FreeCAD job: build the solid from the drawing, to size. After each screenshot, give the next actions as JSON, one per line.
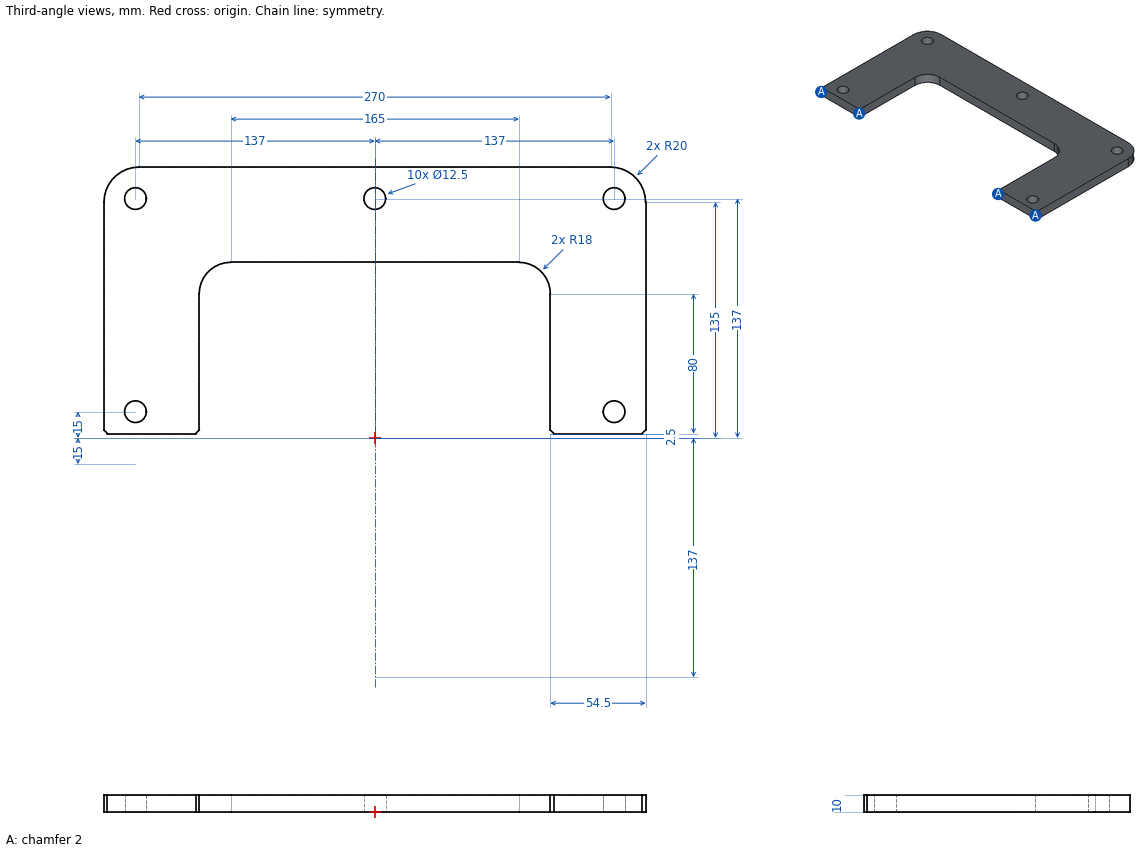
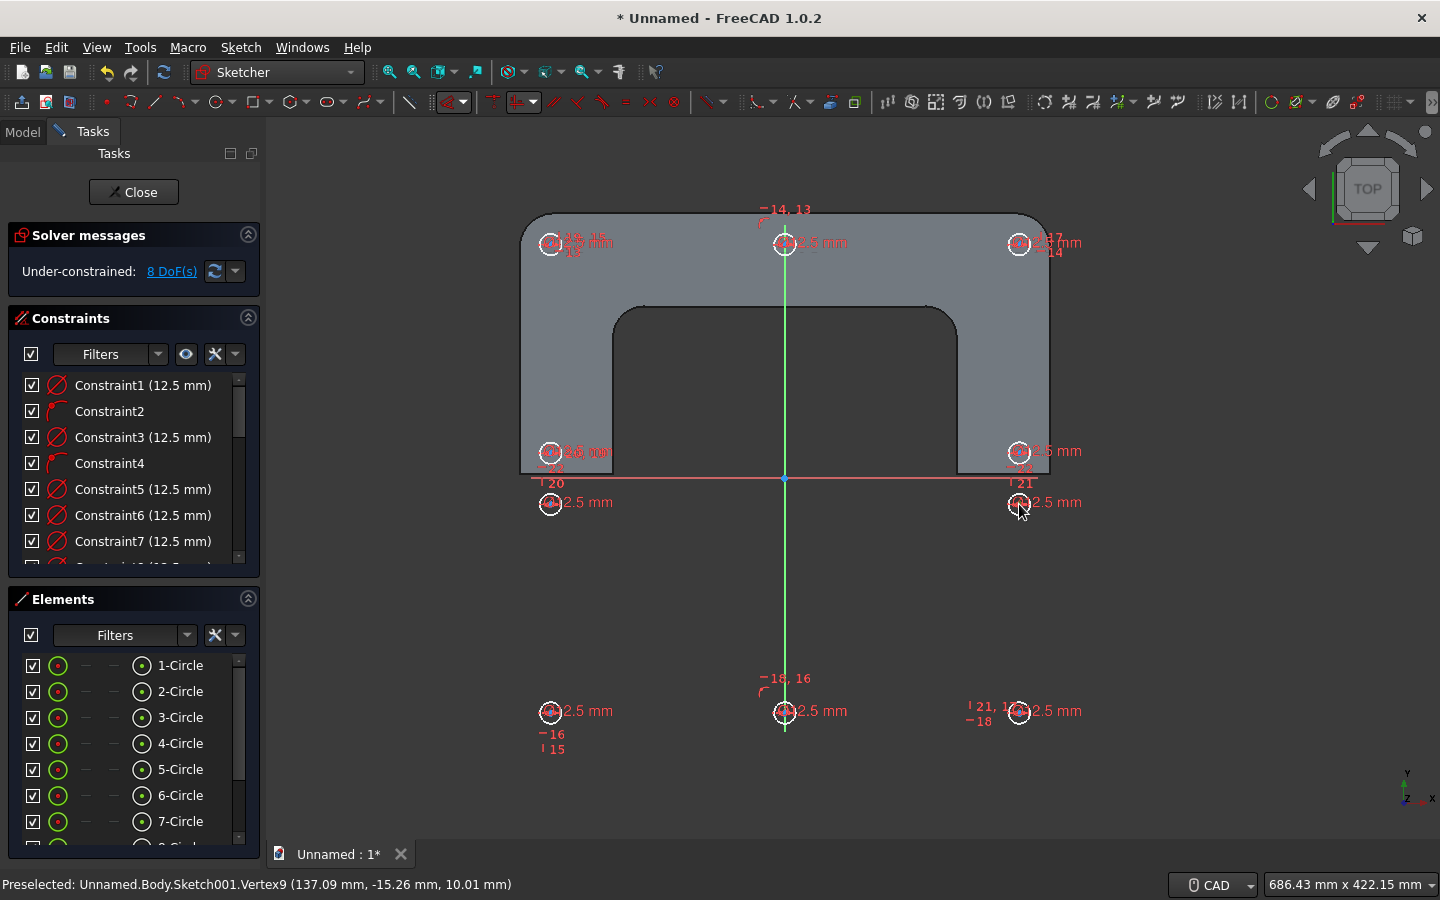
{"action": "left_click", "coordinate": [1019, 453]}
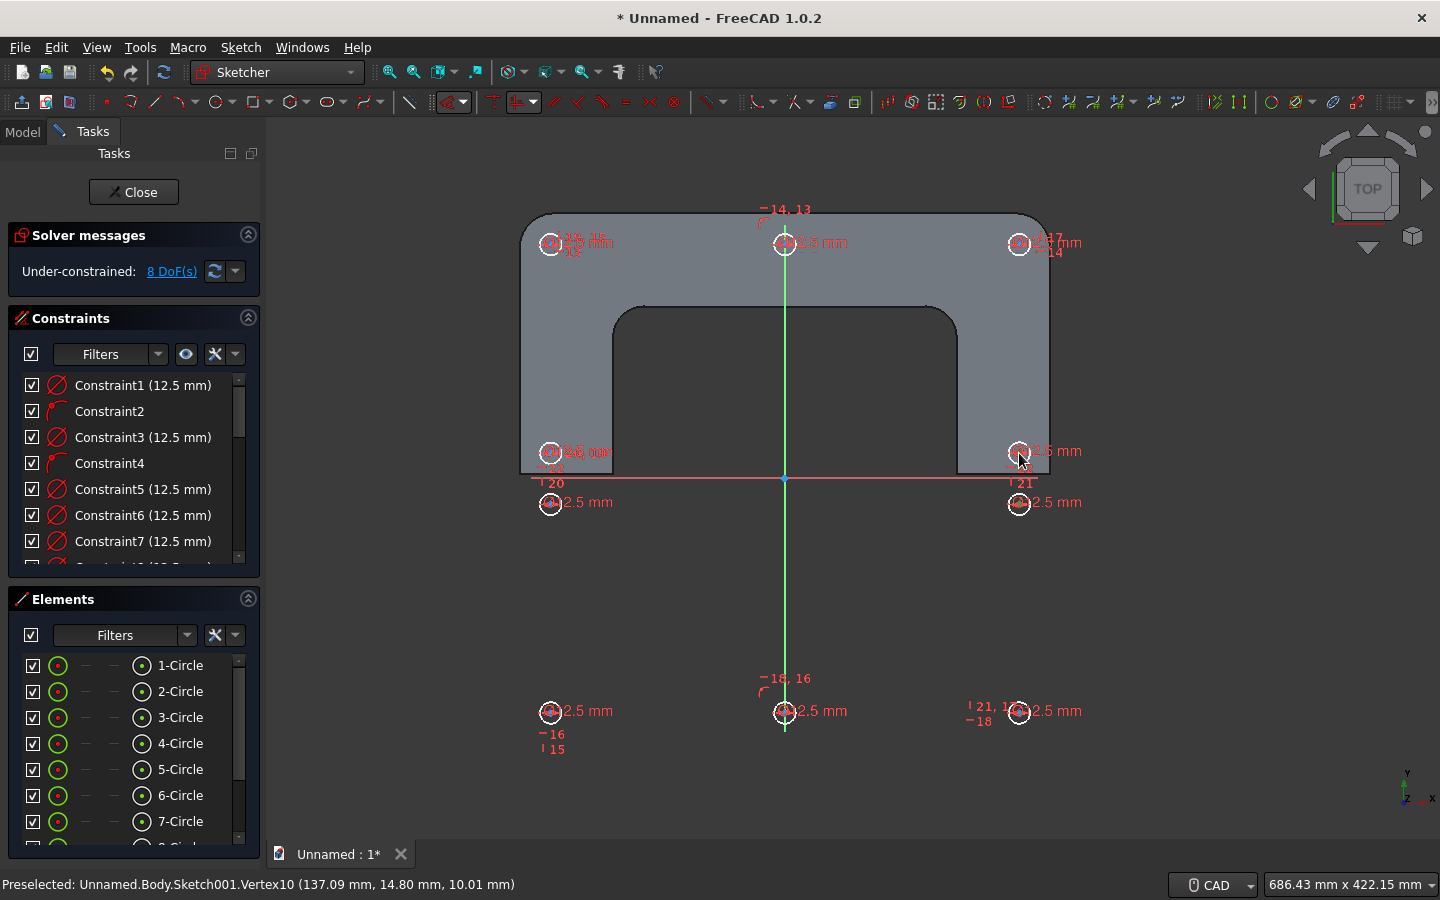
{"action": "key", "text": "v"}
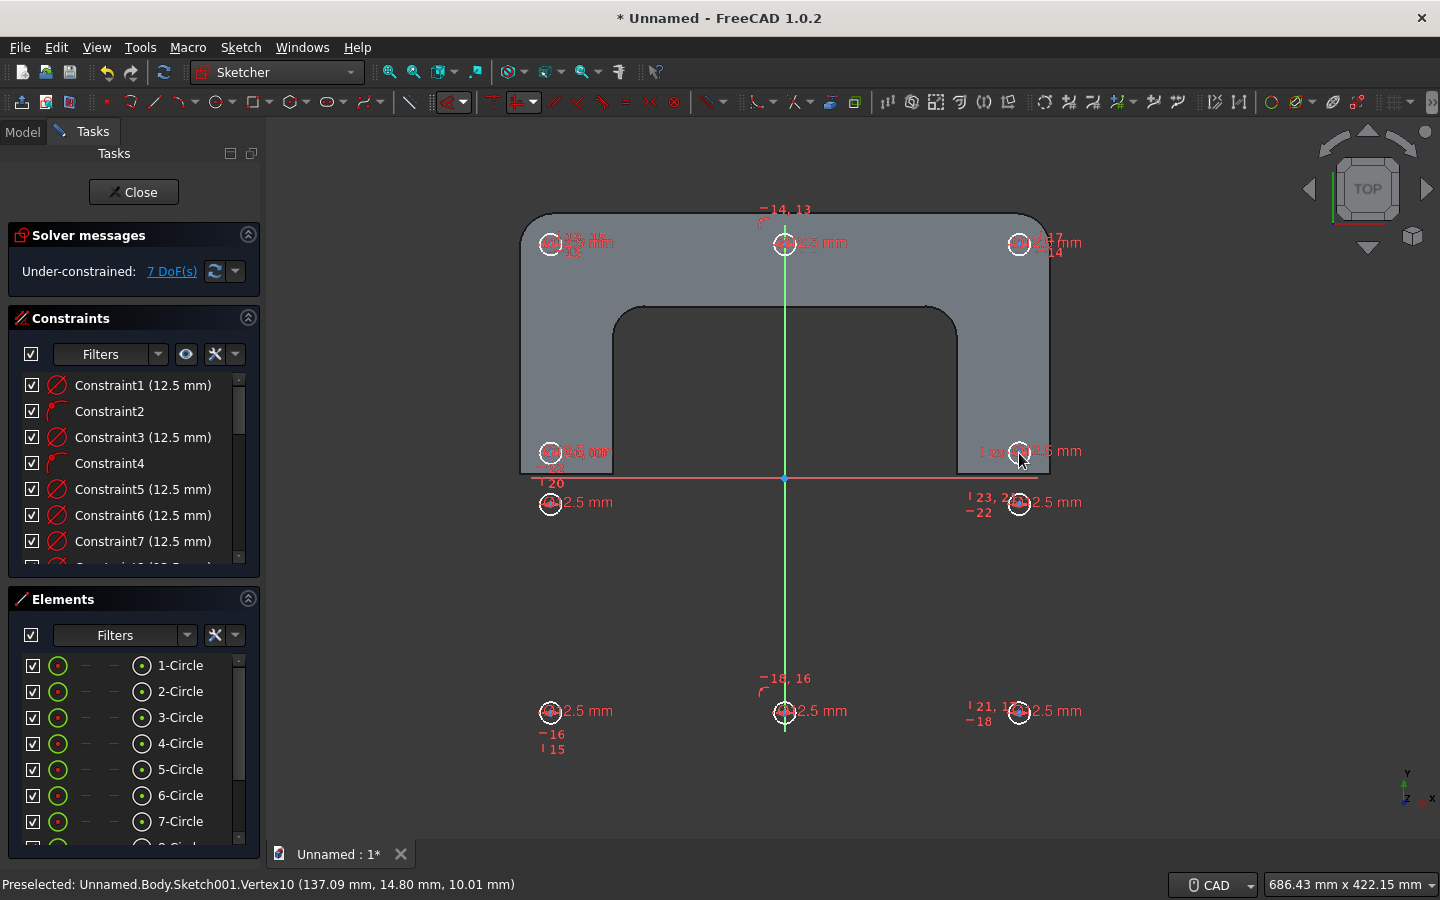
{"action": "left_click", "coordinate": [551, 453]}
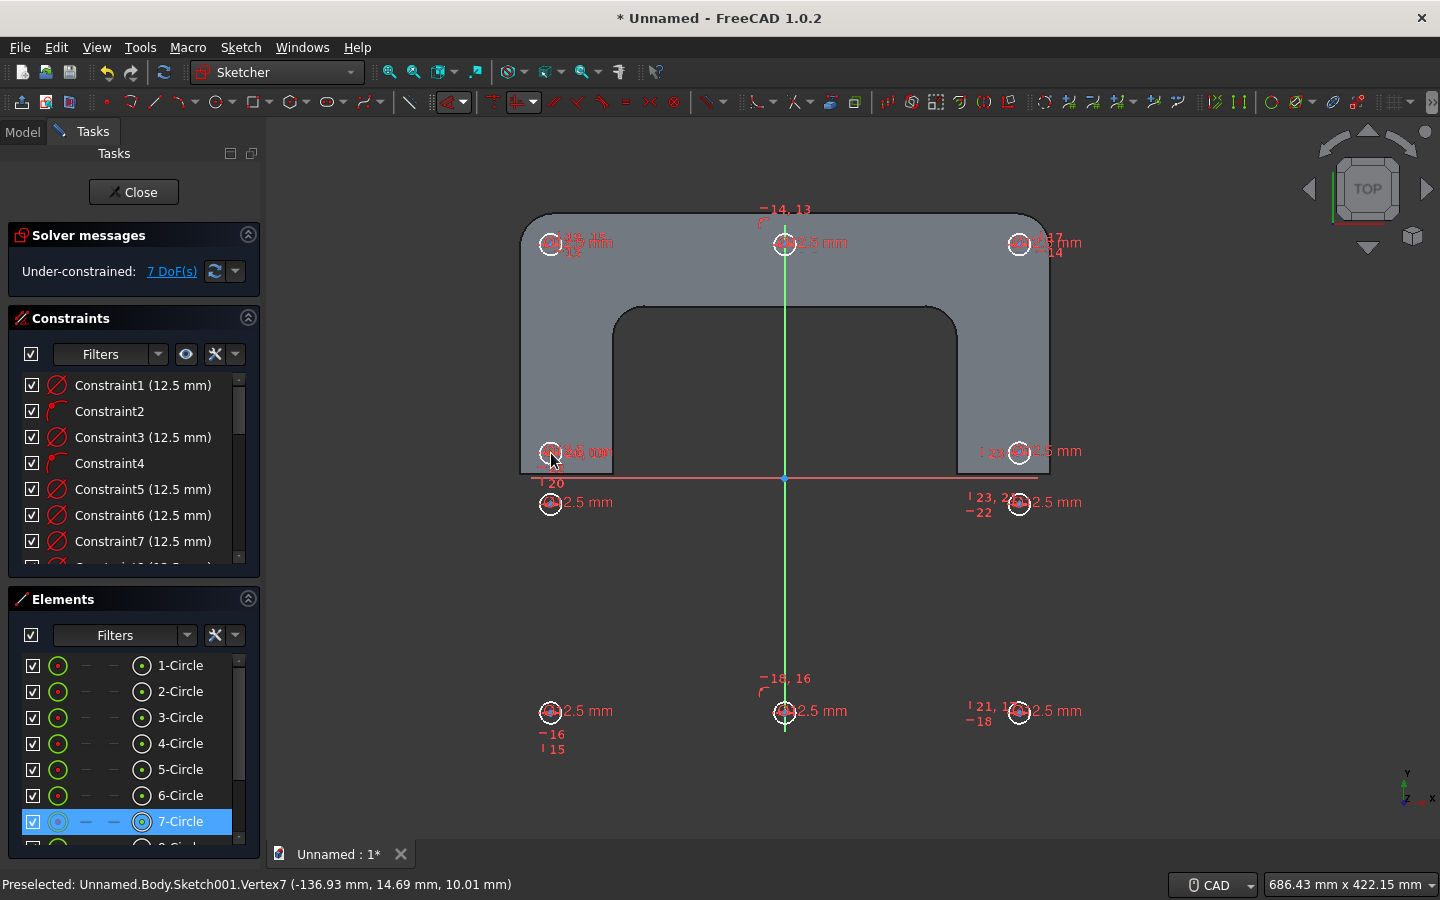
{"action": "left_click", "coordinate": [1019, 453]}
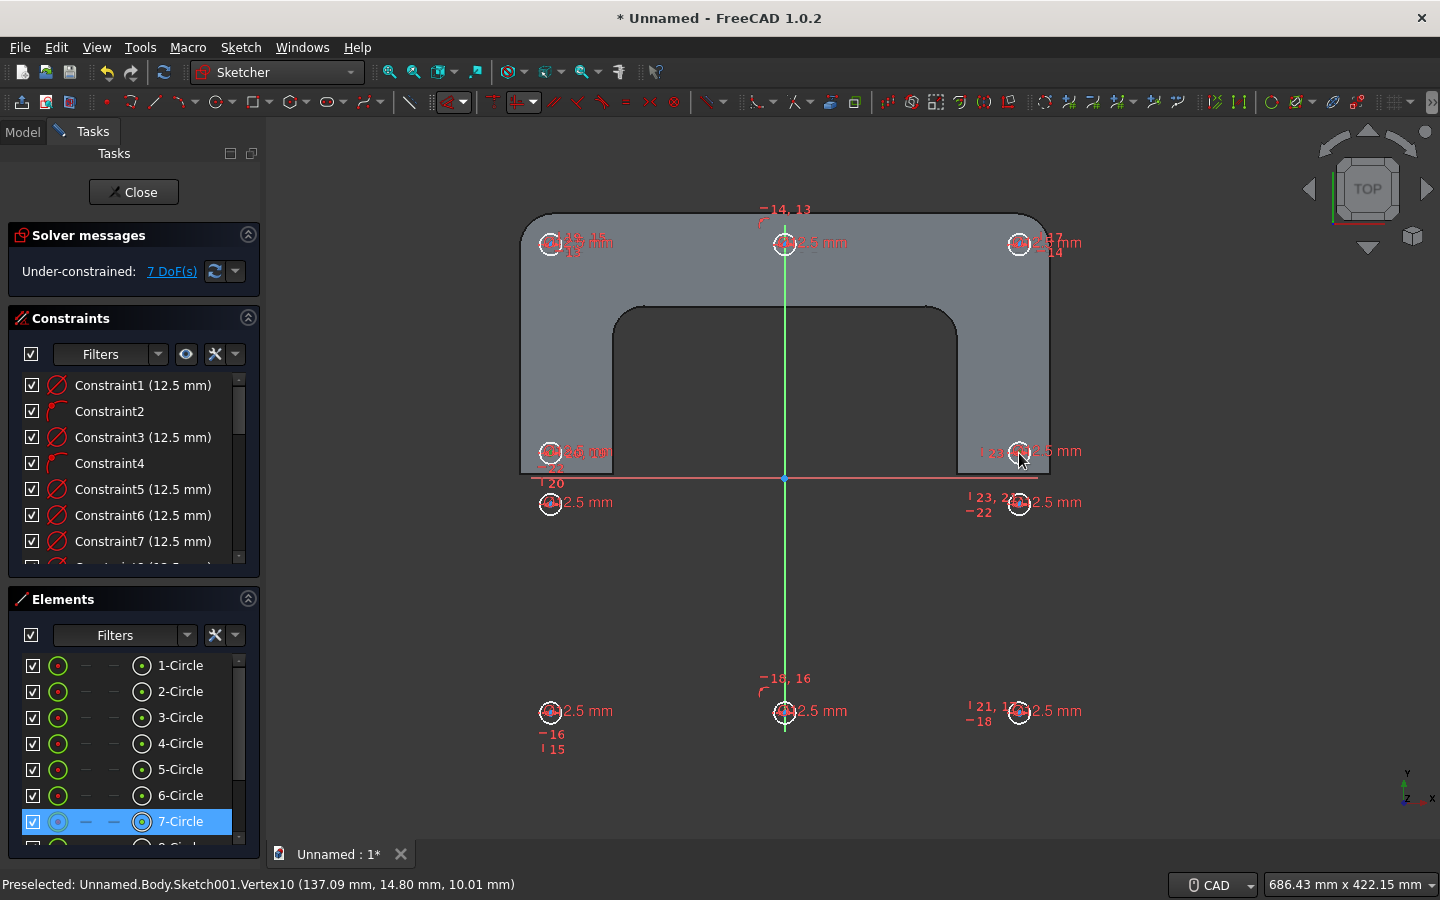
{"action": "key", "text": "h"}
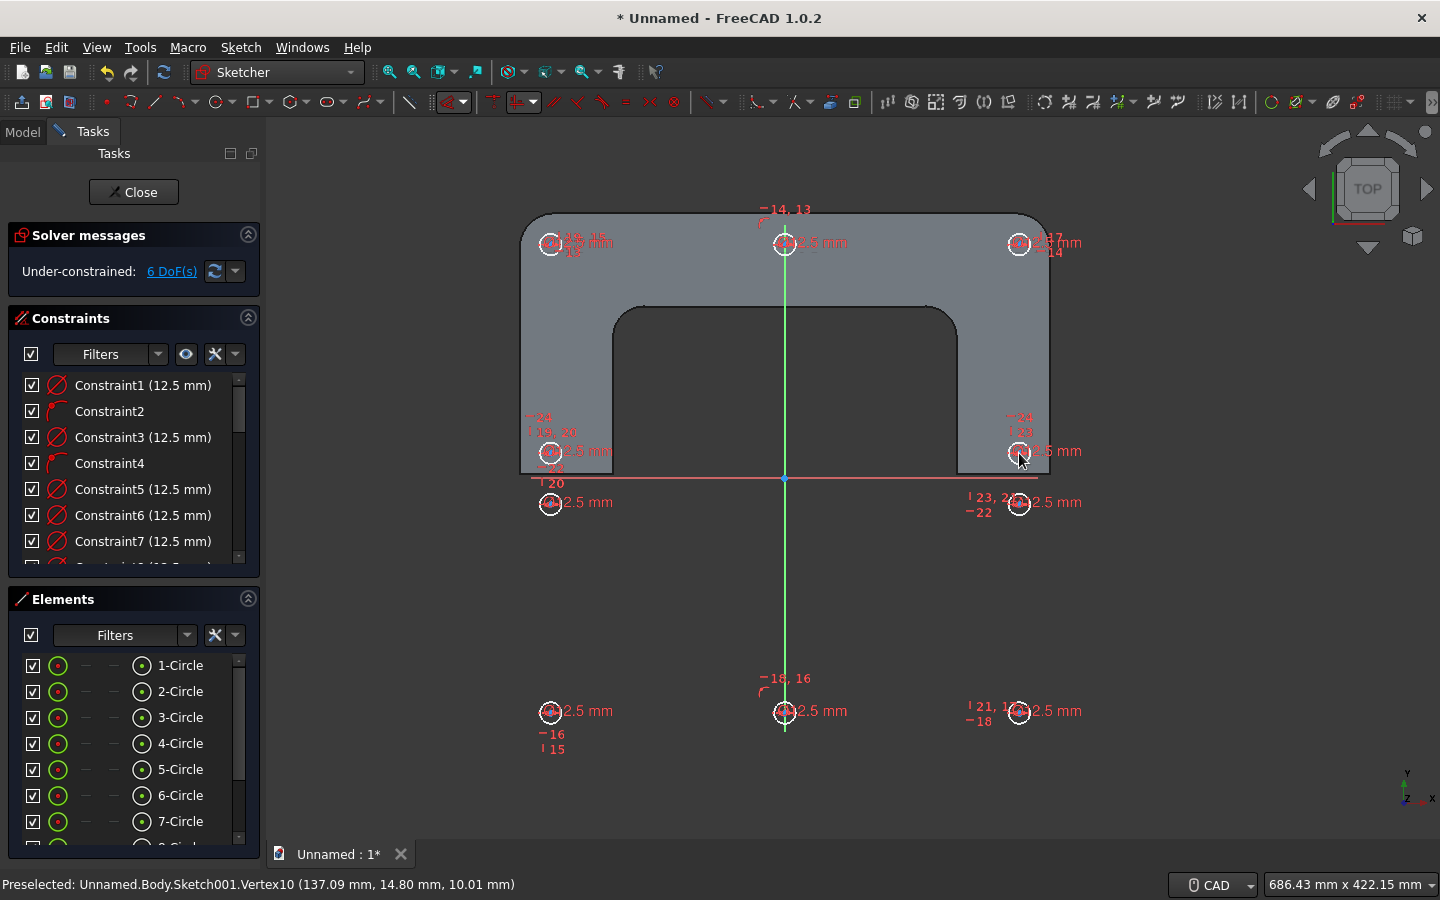
{"action": "scroll", "coordinate": [551, 453], "scroll_direction": "up", "scroll_amount": 3}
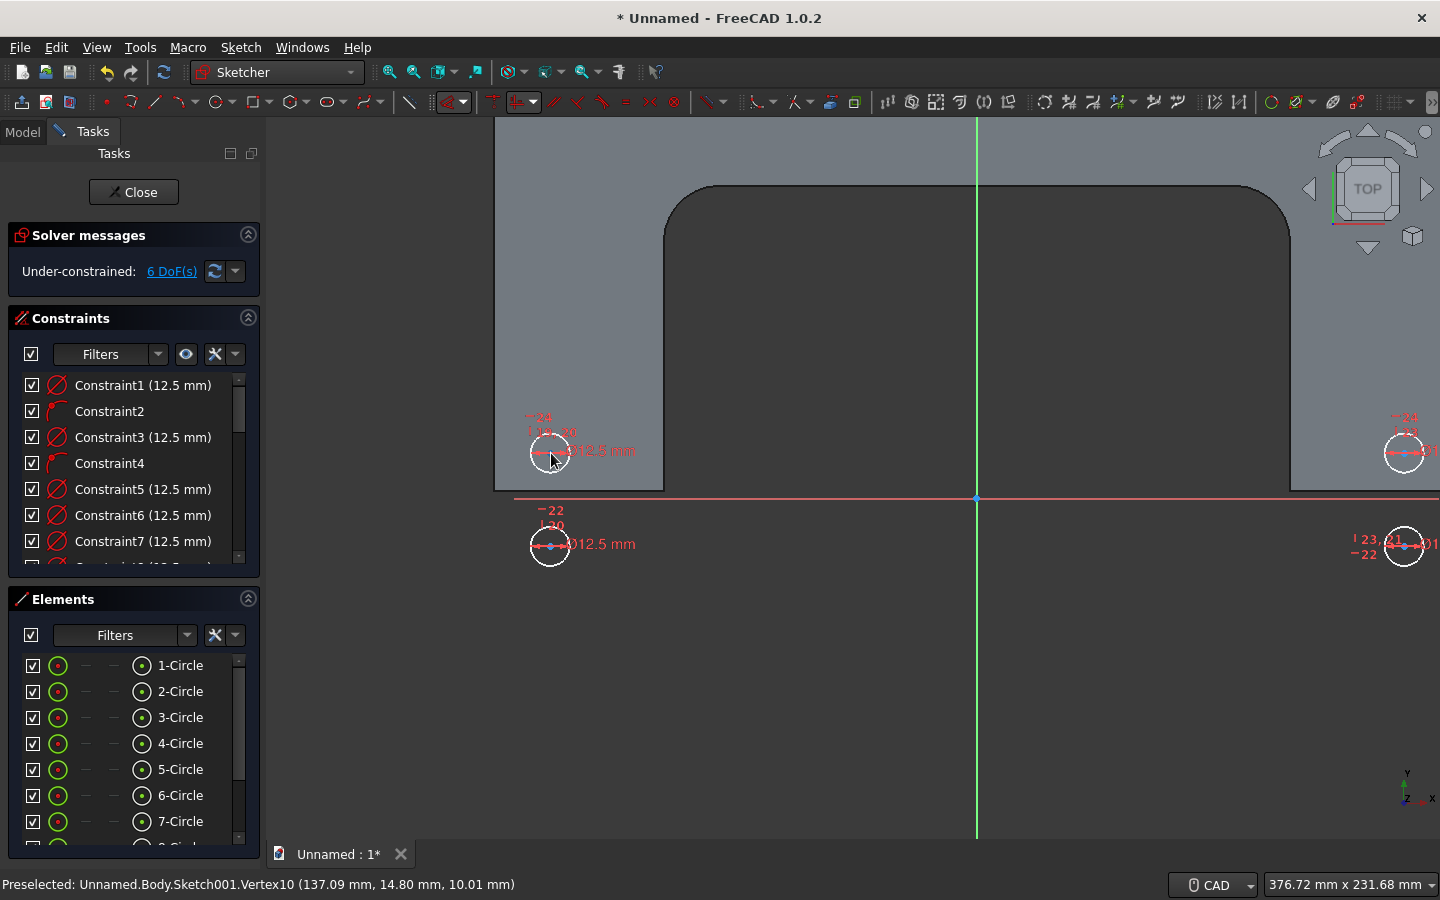
{"action": "left_click", "coordinate": [550, 453]}